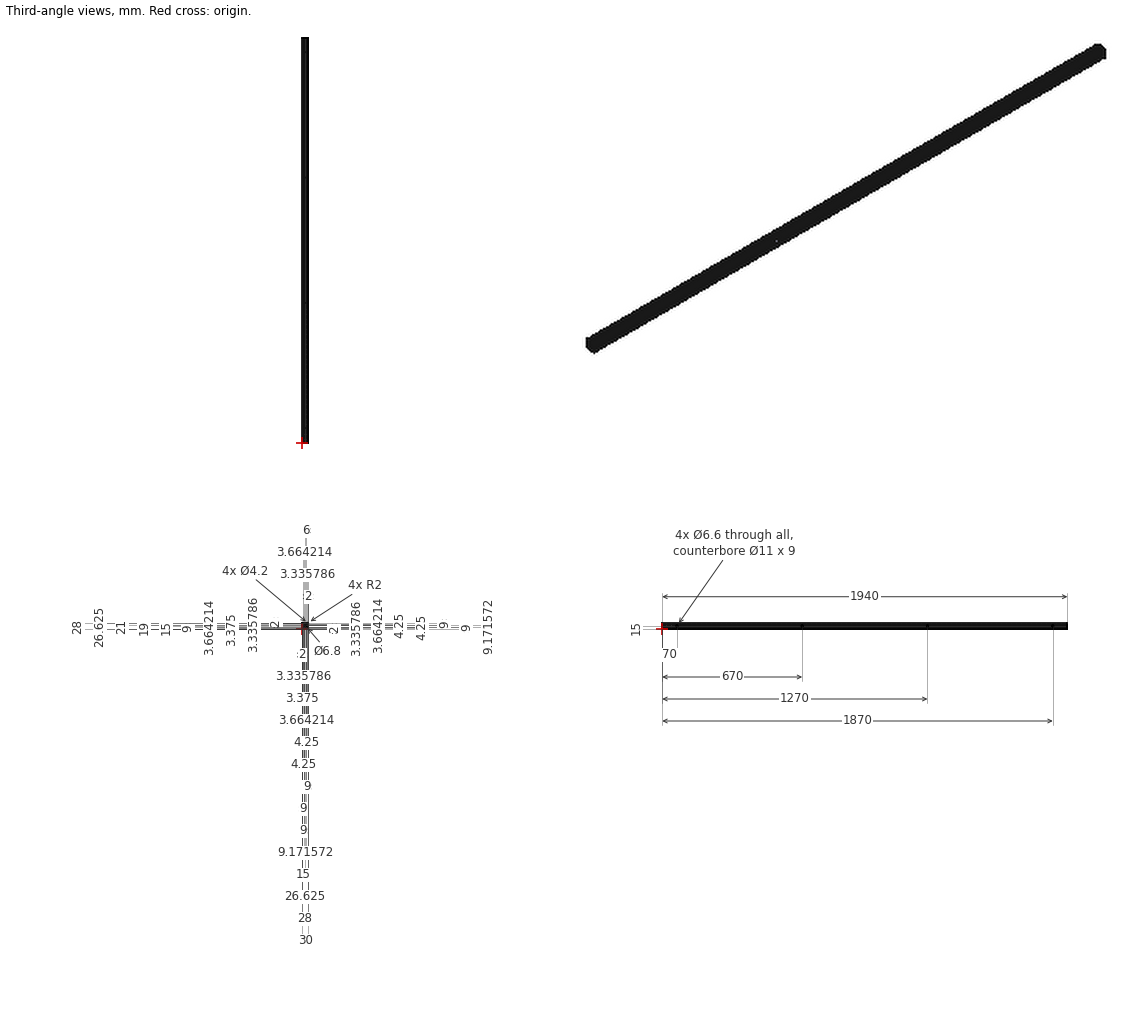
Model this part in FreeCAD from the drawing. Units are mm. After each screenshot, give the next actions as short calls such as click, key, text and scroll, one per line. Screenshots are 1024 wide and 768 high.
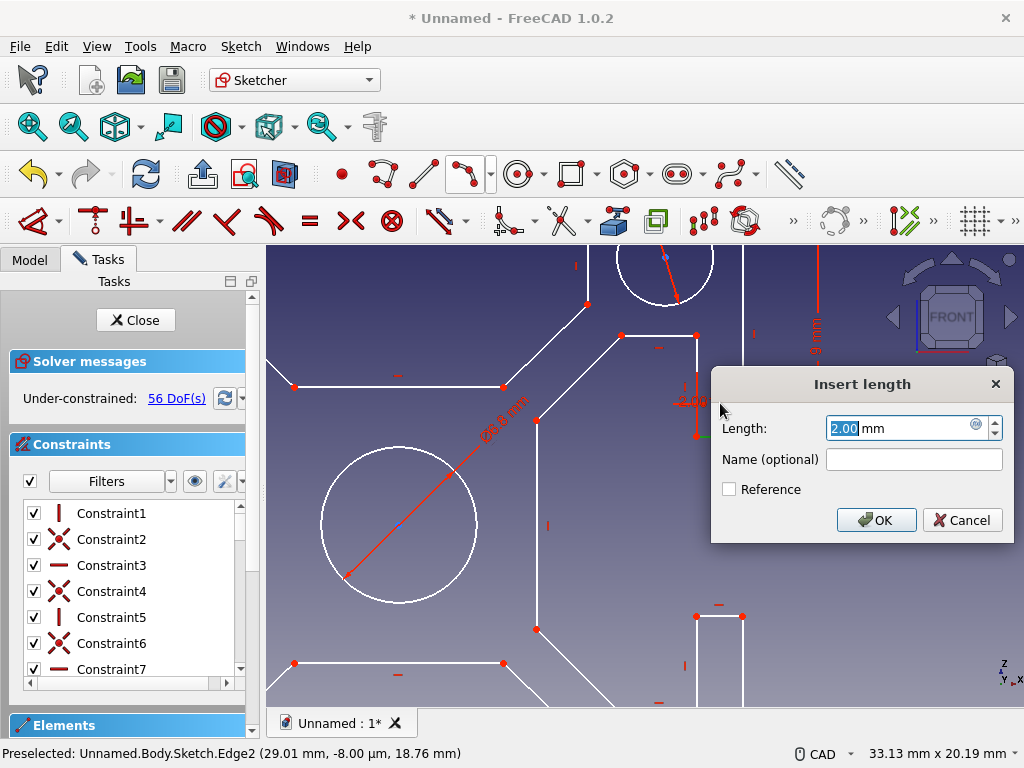
text(2)
key(Return)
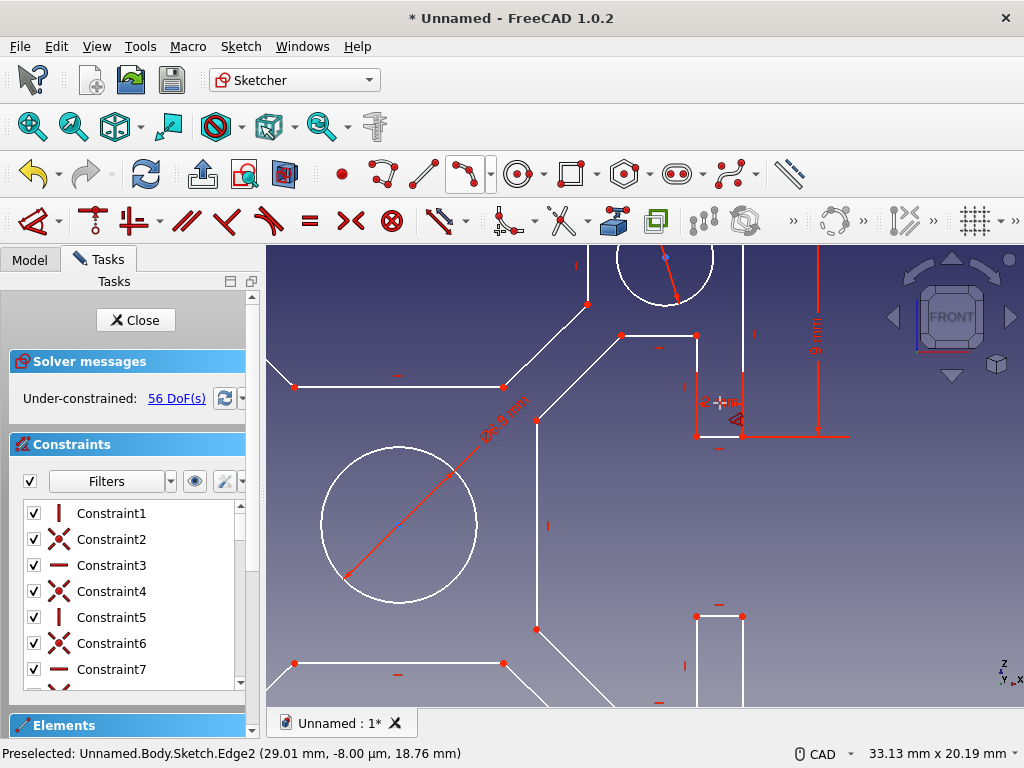
click(711, 616)
click(720, 650)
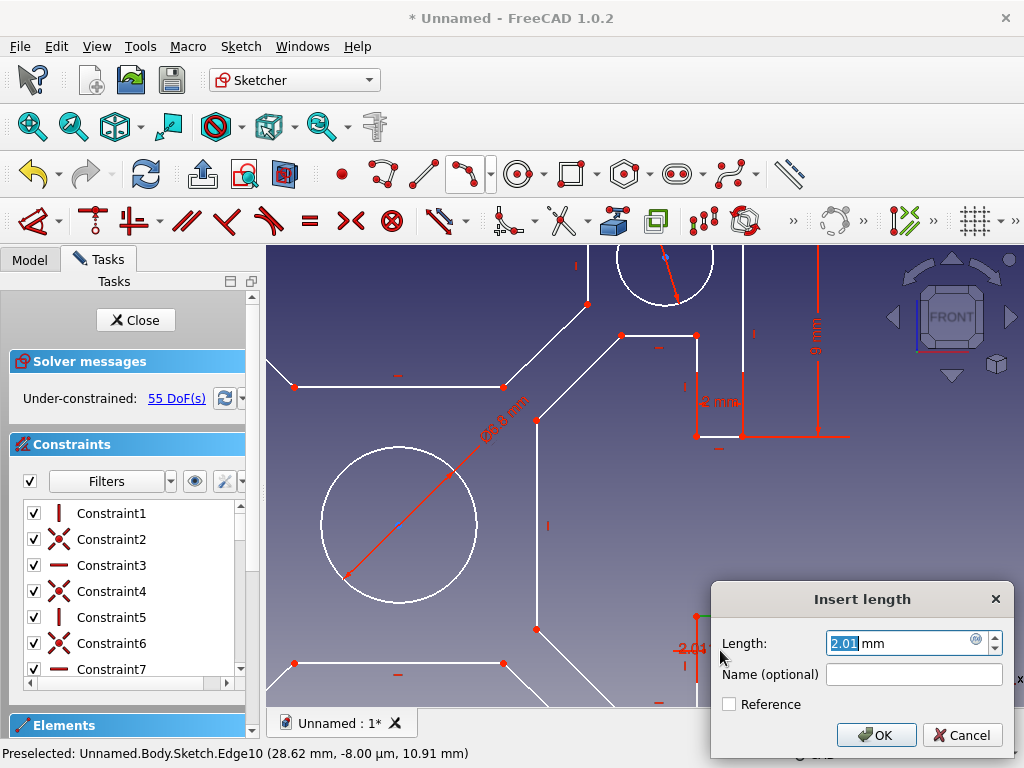
text(2)
key(Return)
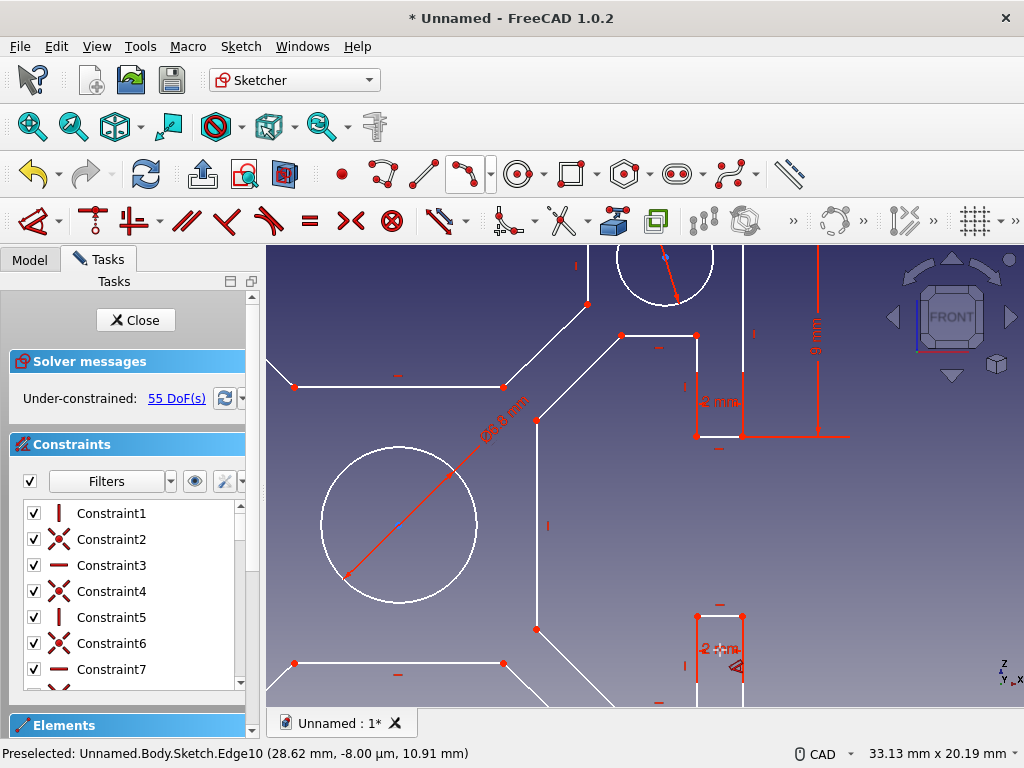
click(743, 677)
click(777, 626)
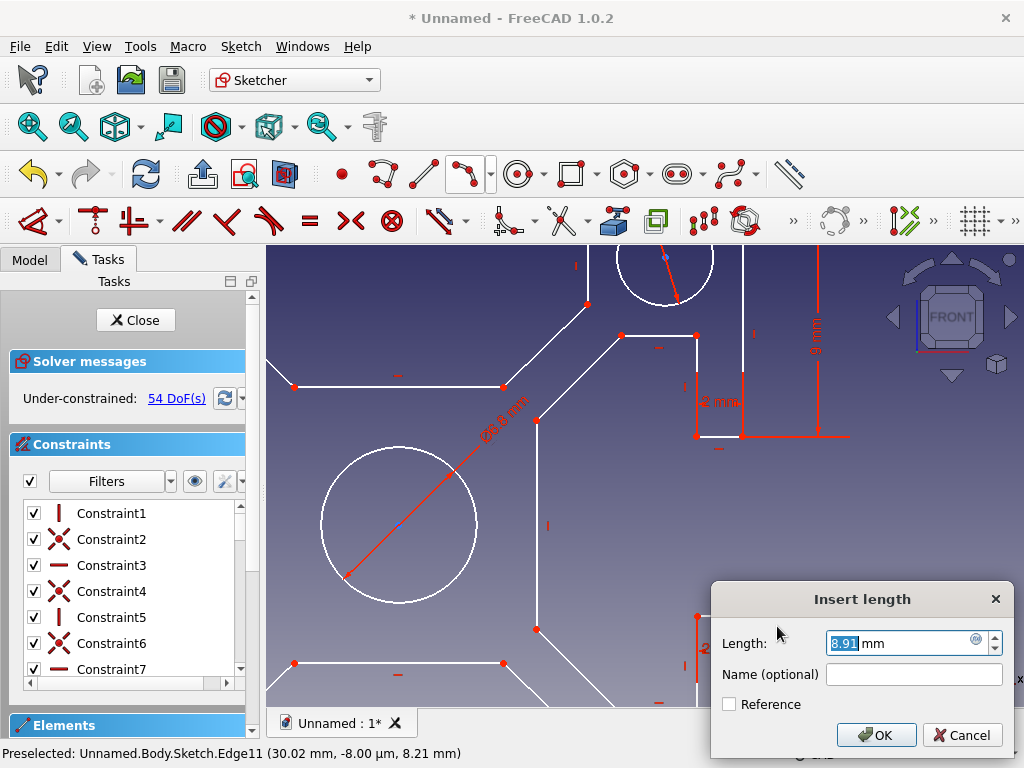
text(9)
key(Return)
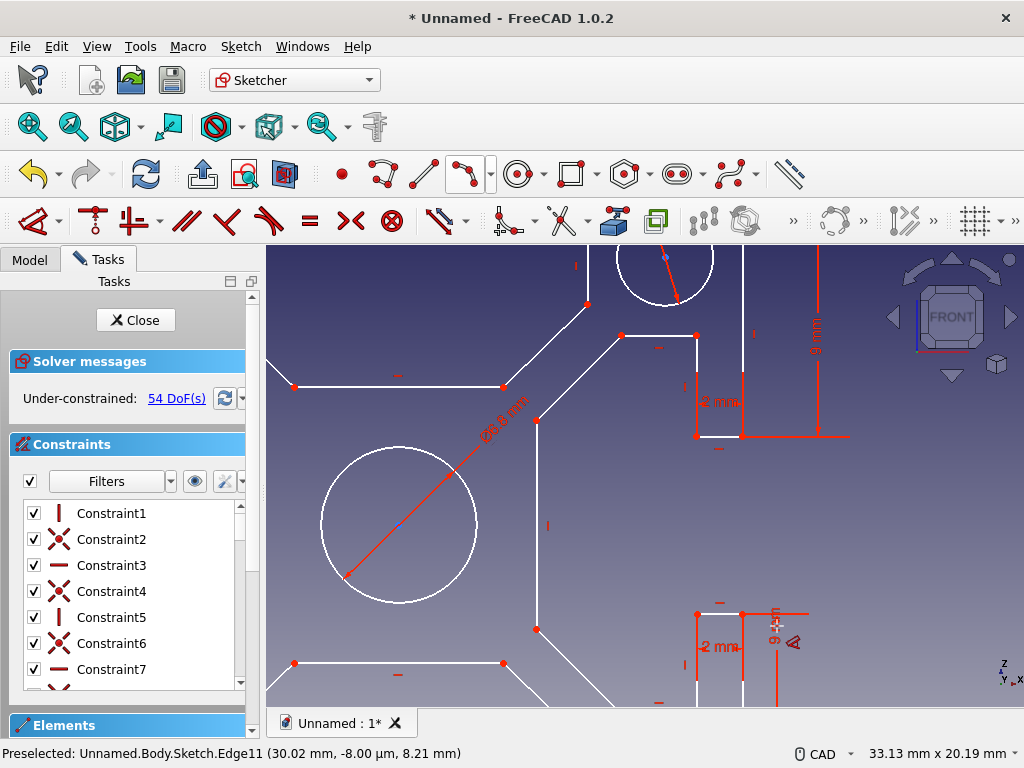
scroll(721, 438, down, 4)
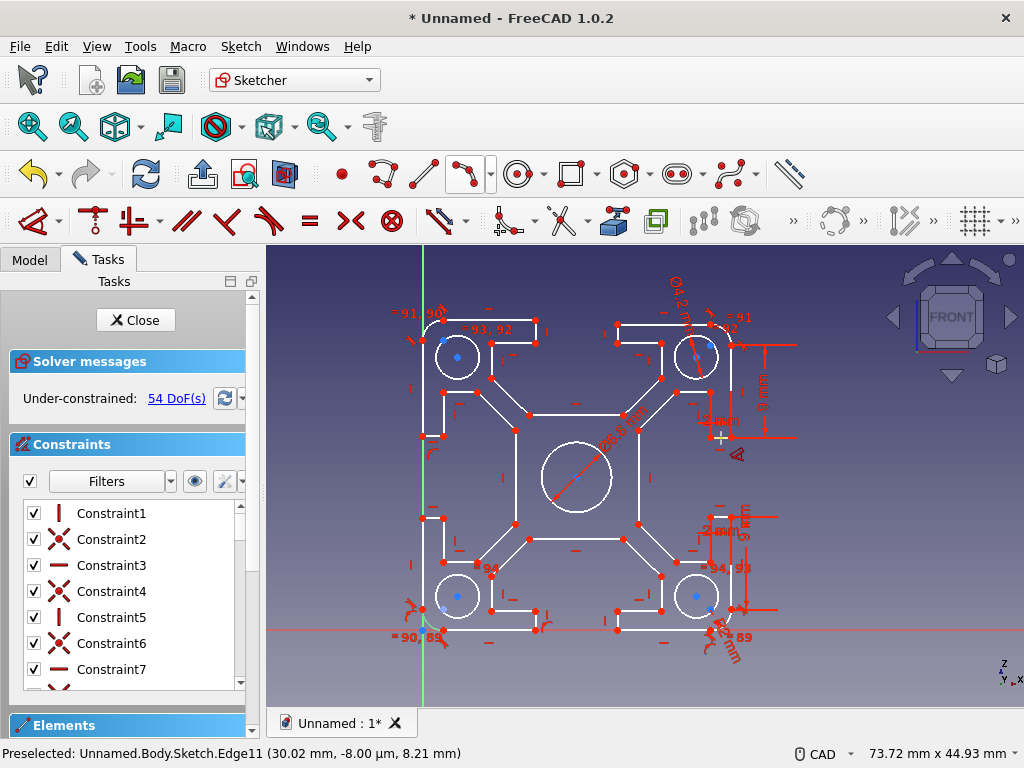
click(683, 630)
click(664, 664)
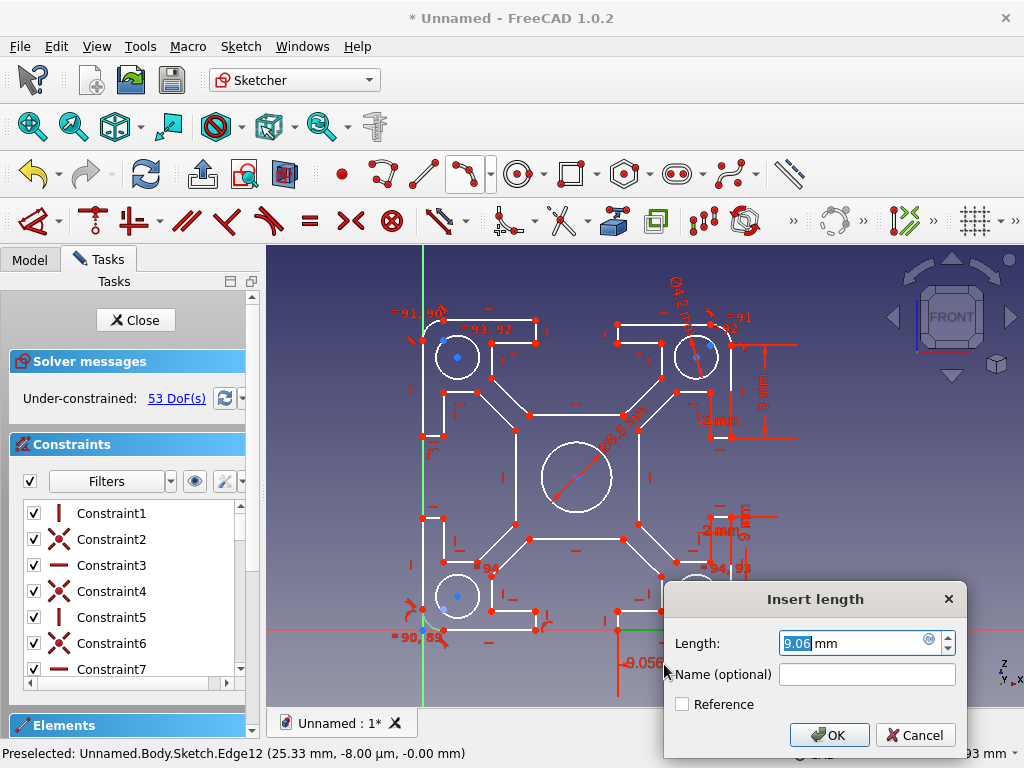
text(9)
key(Return)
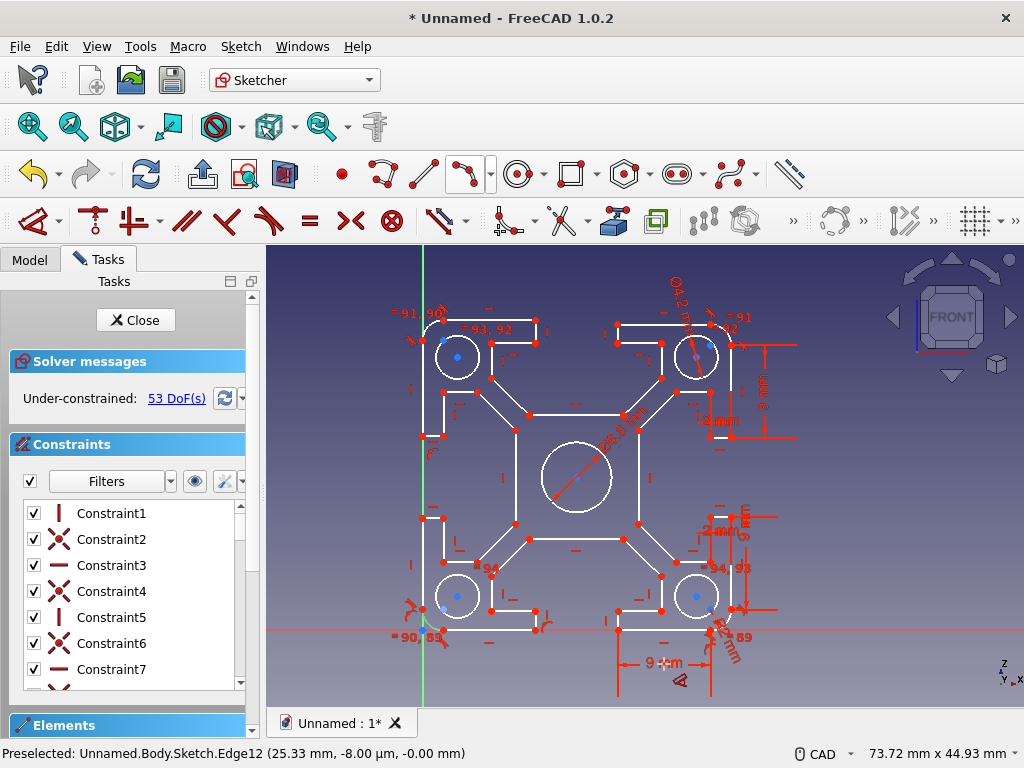
scroll(618, 621, up, 4)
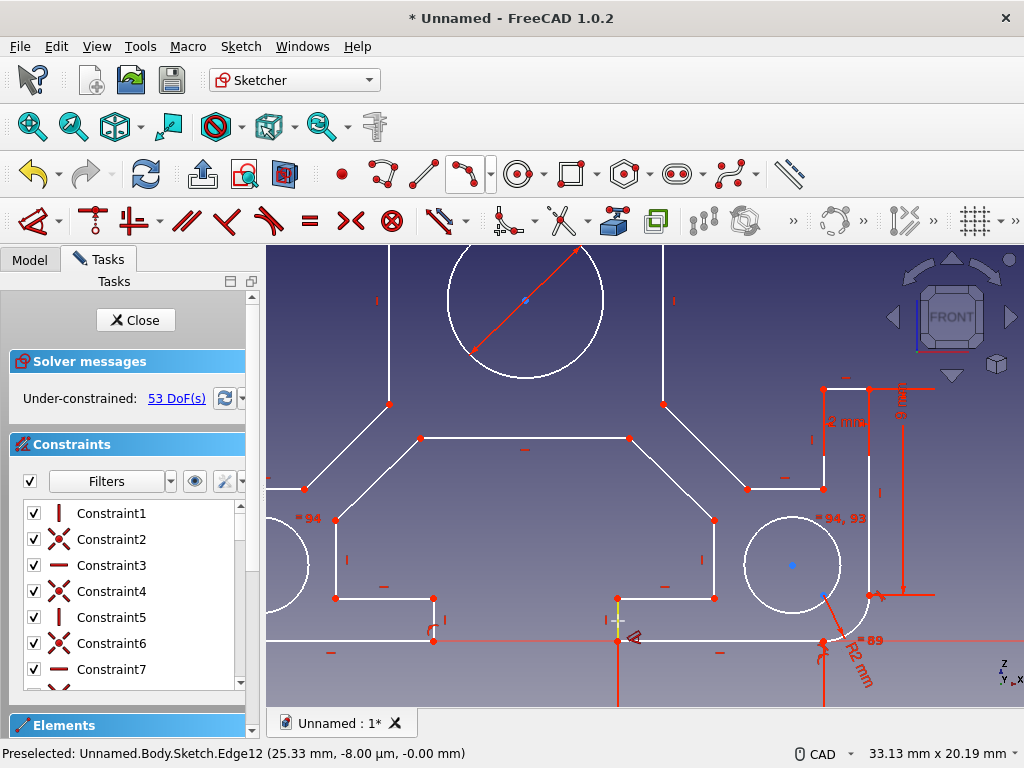
click(618, 620)
click(652, 620)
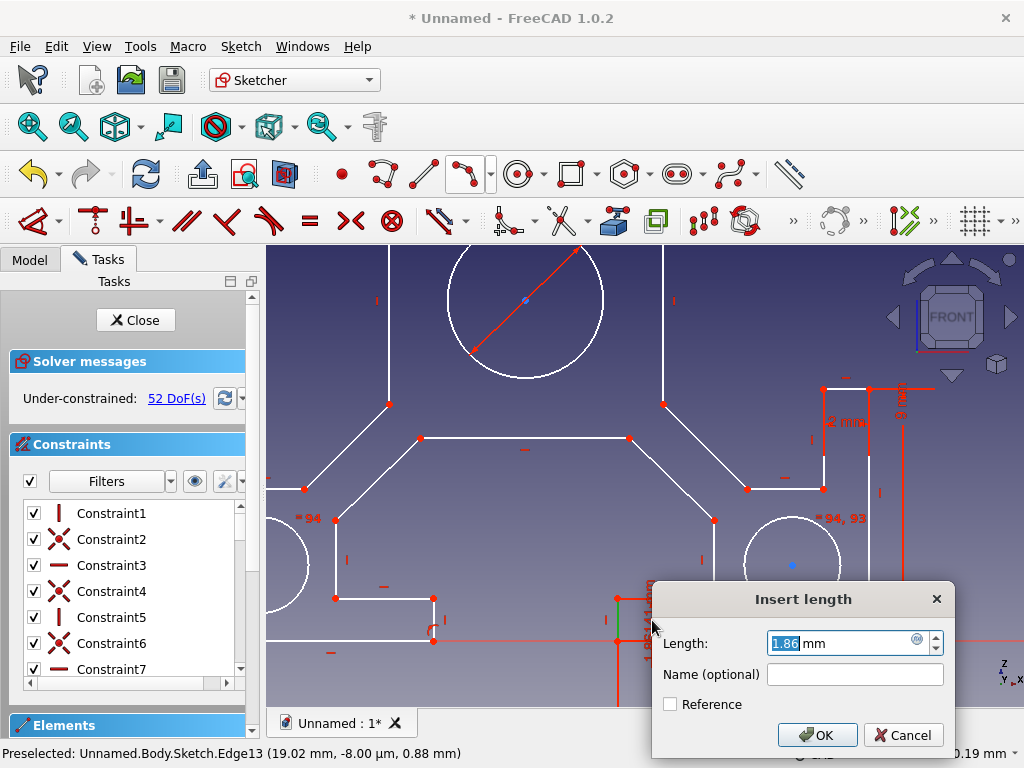
text(2)
key(Return)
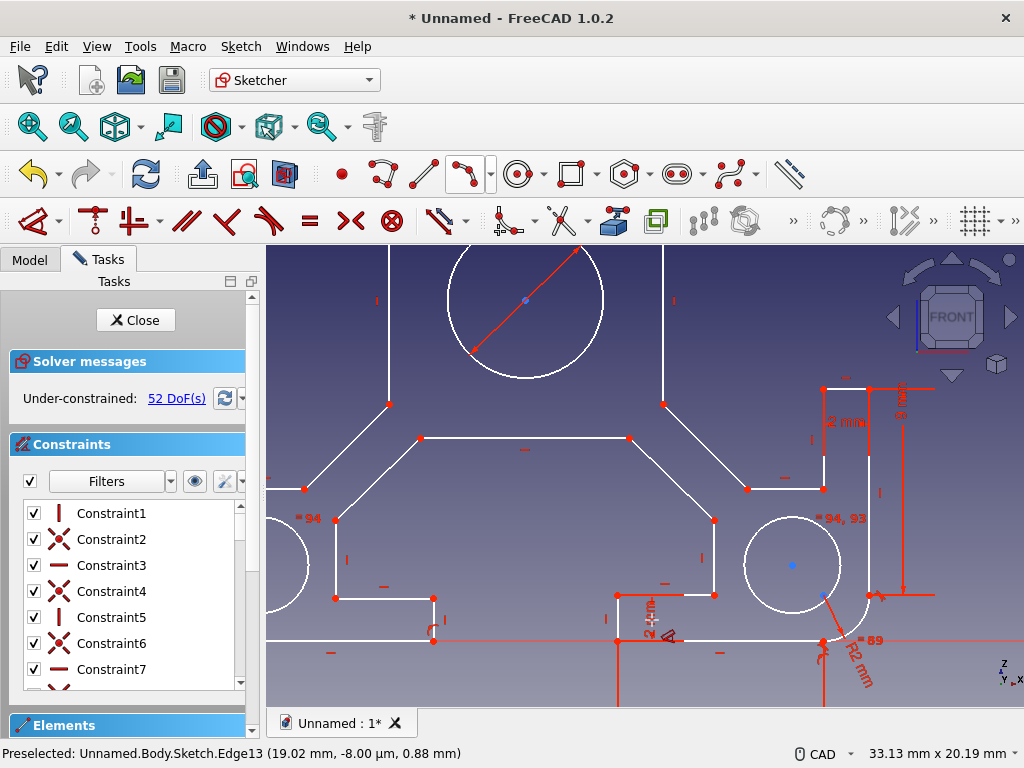
click(434, 611)
click(400, 620)